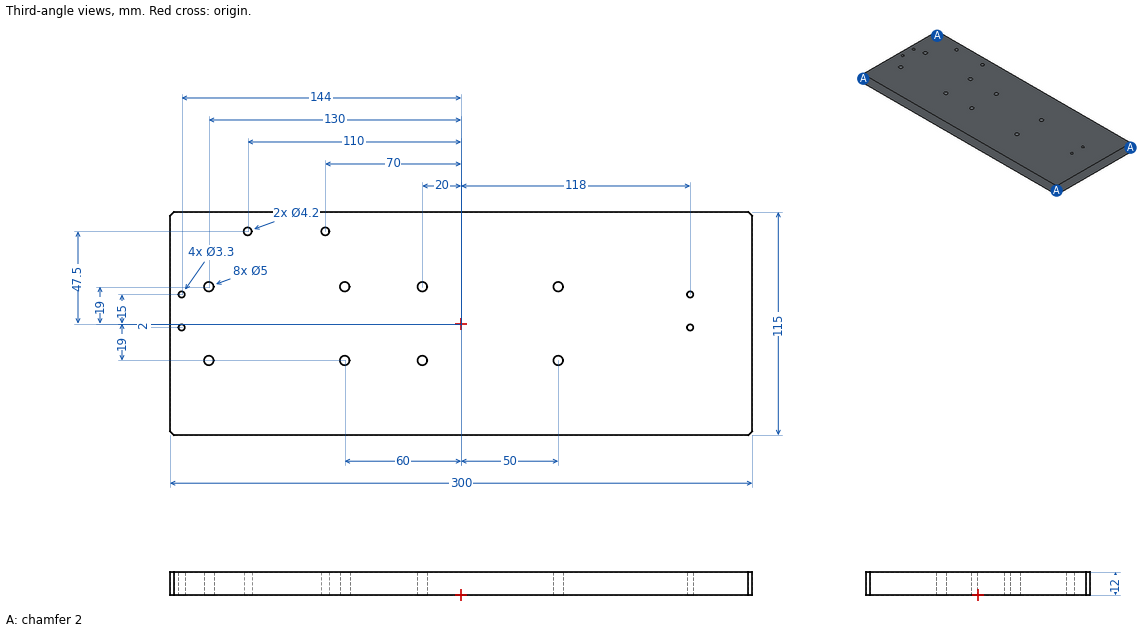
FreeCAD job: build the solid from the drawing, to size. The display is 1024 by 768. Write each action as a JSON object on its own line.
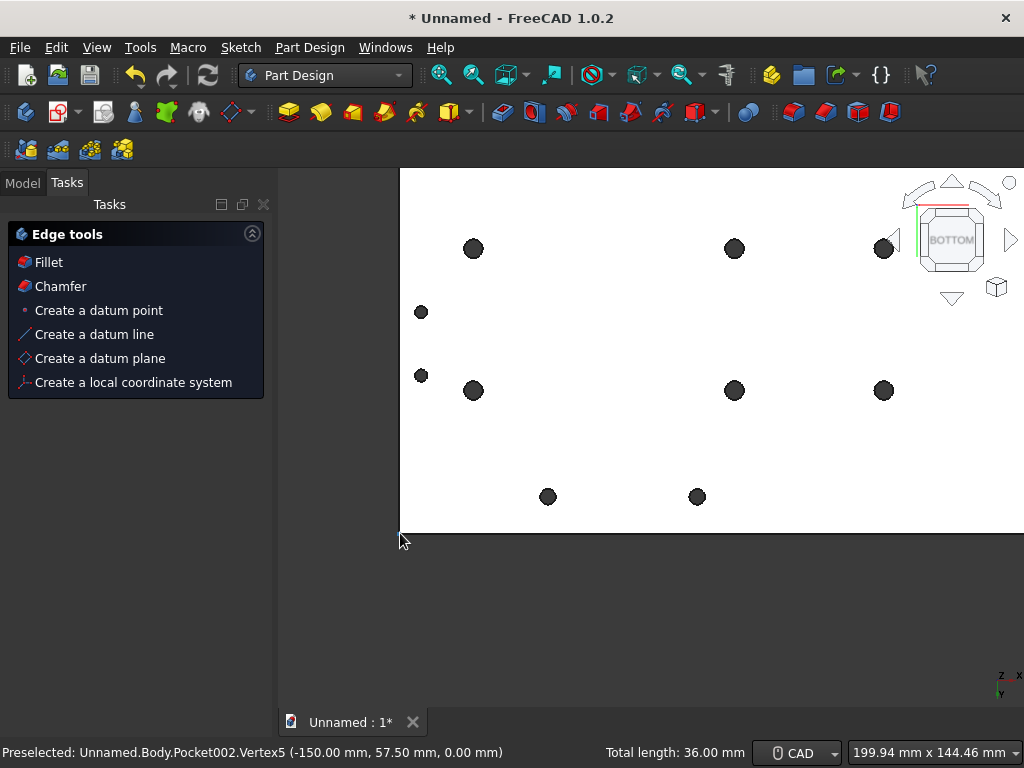
{"action": "key", "text": "v f"}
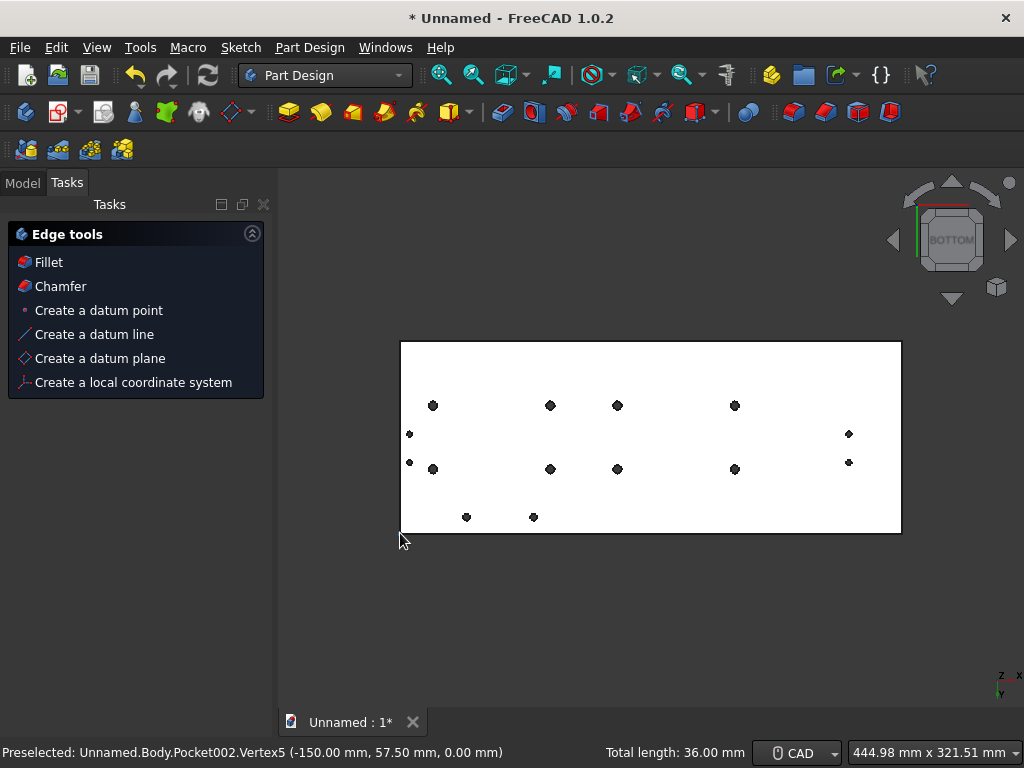
{"action": "key", "text": "4"}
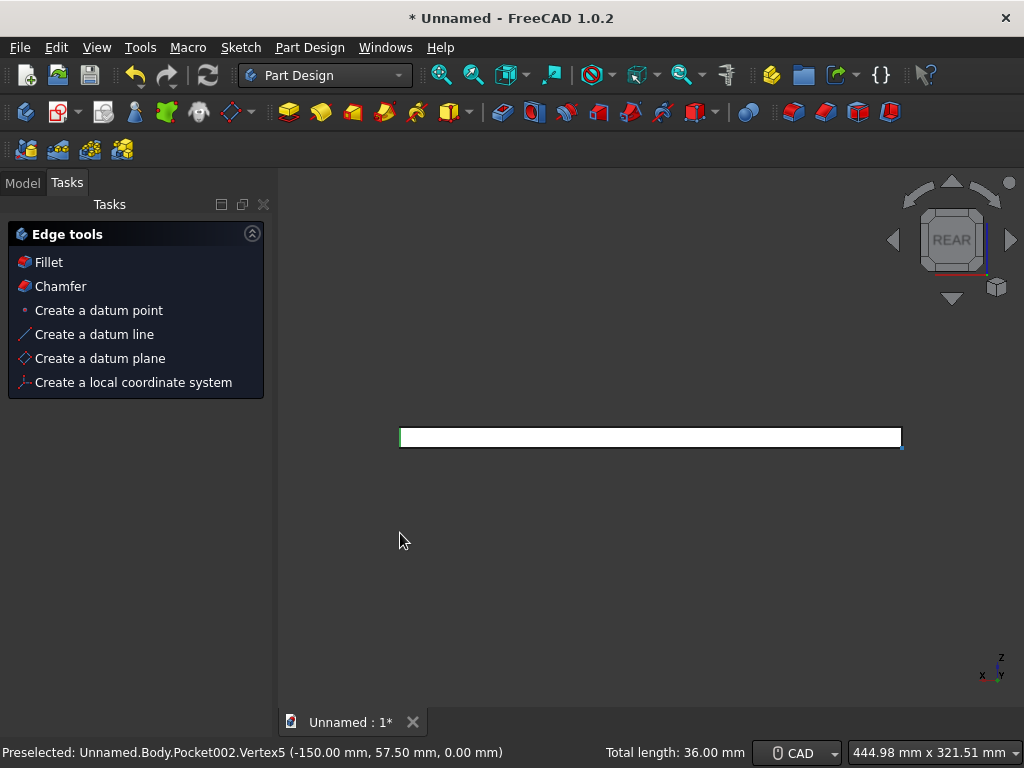
{"action": "left_click", "coordinate": [902, 436], "text": "ctrl"}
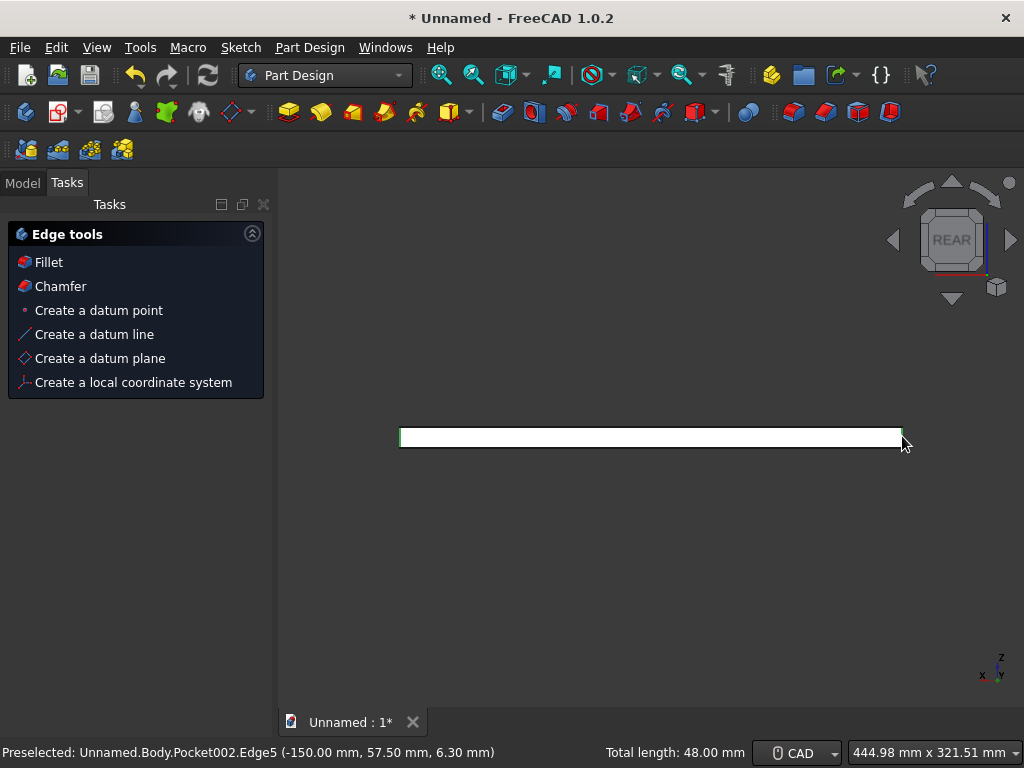
{"action": "left_click", "coordinate": [826, 112]}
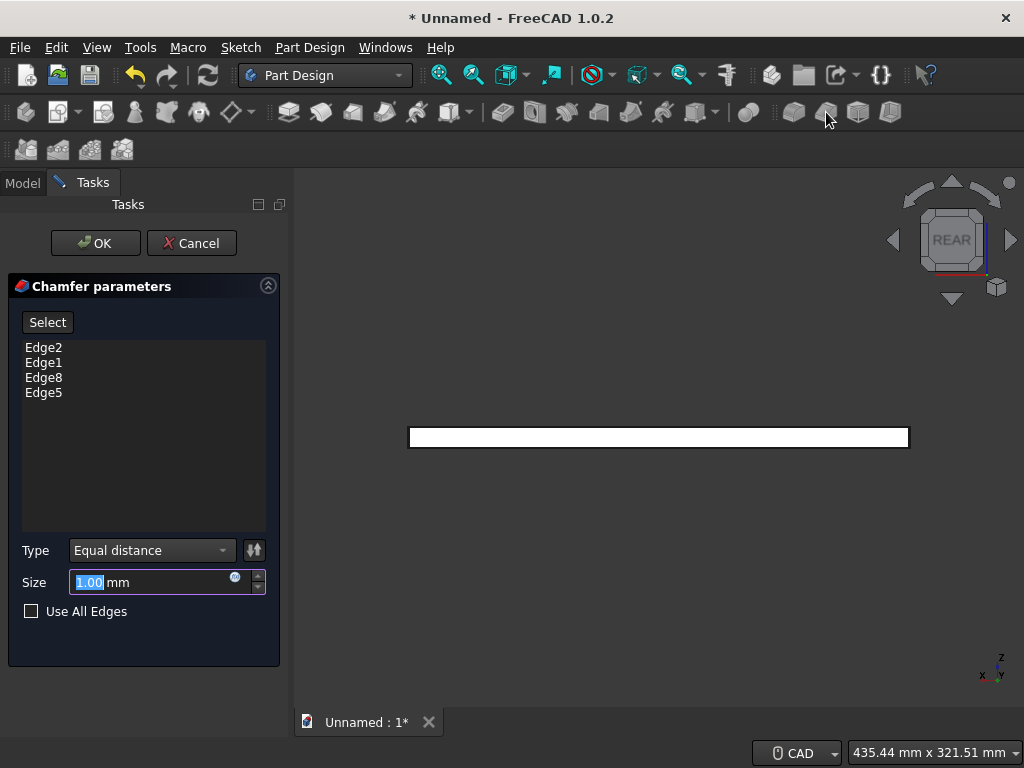
{"action": "type", "text": "2"}
{"action": "key", "text": "Tab"}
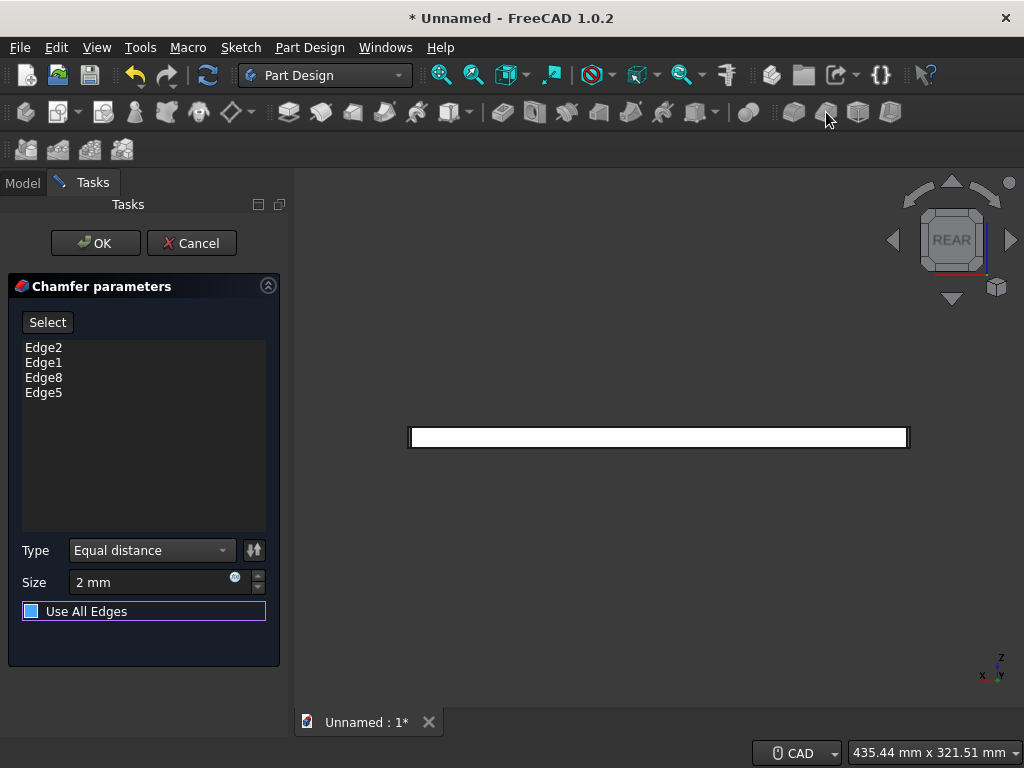
{"action": "left_click", "coordinate": [96, 243]}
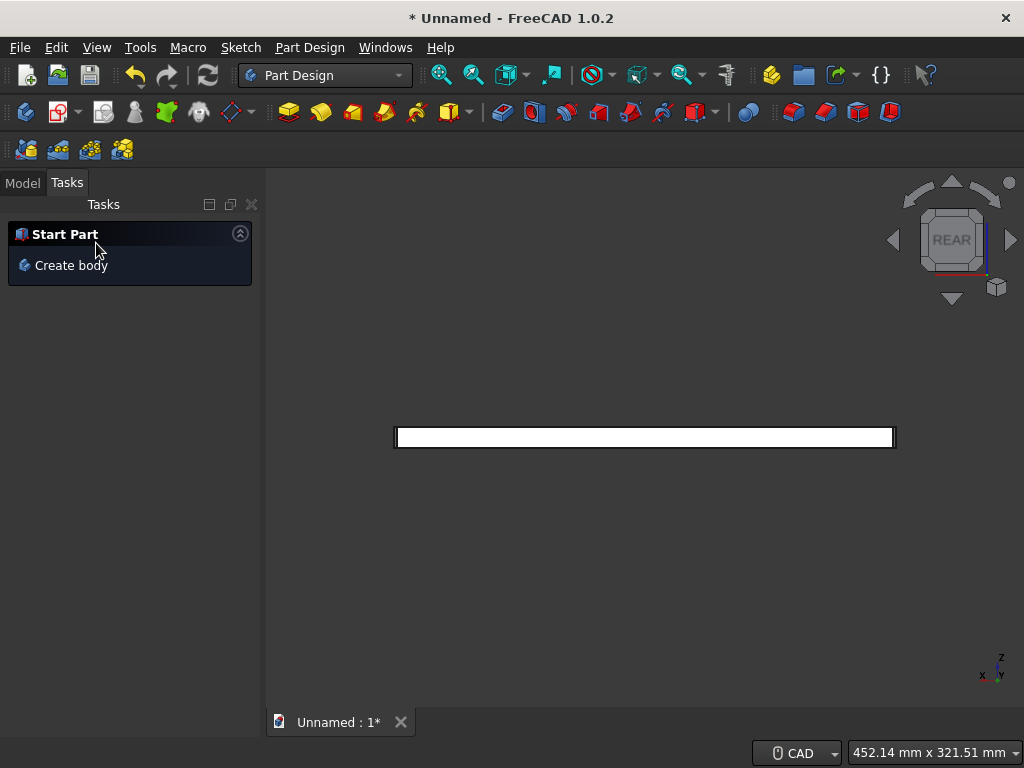
{"action": "key", "text": "0"}